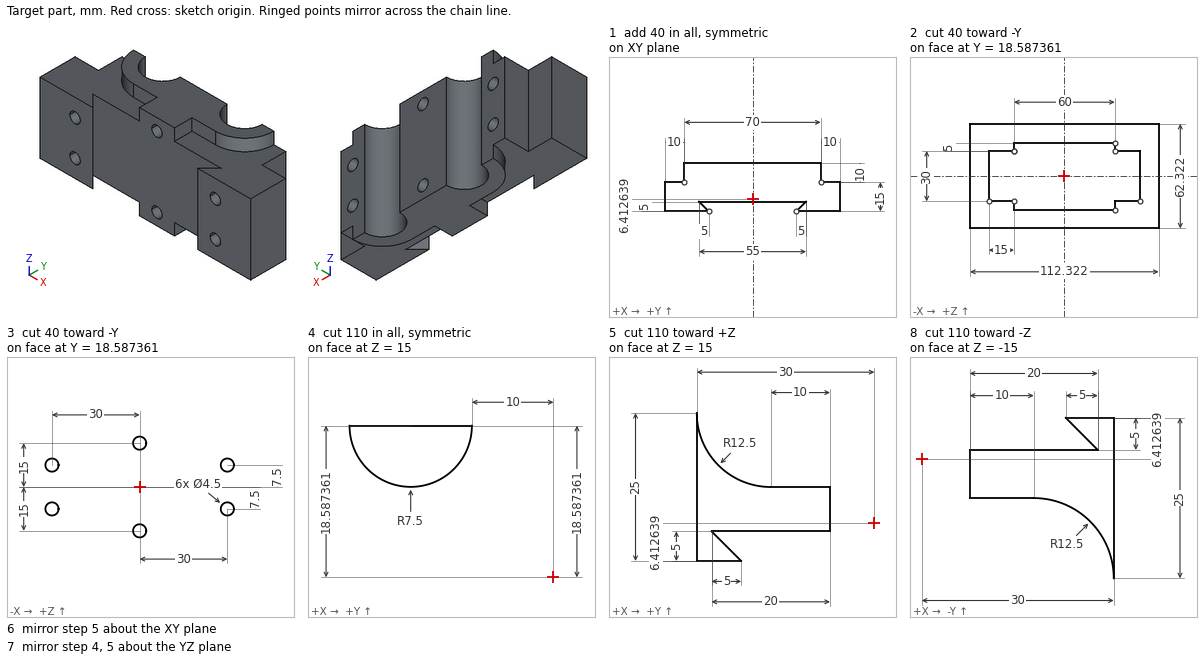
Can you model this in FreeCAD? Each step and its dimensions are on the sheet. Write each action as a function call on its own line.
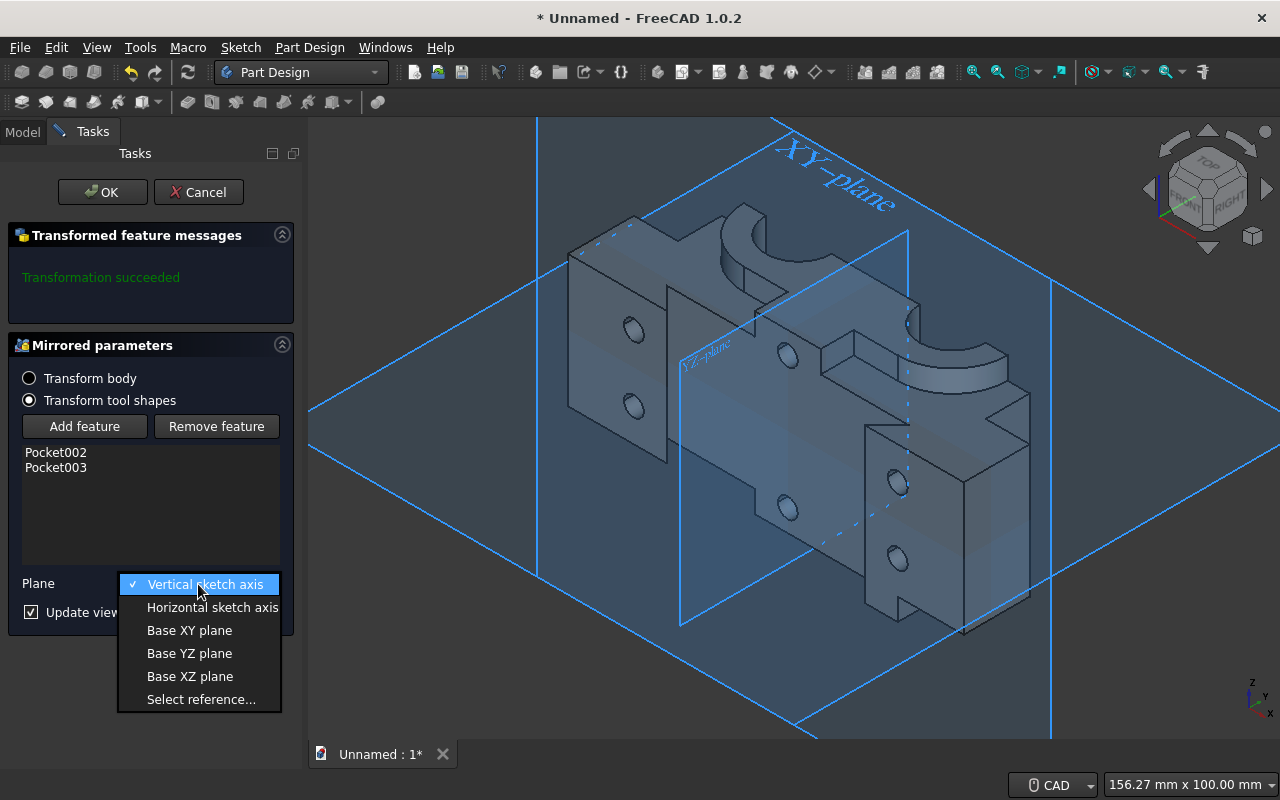
click(198, 654)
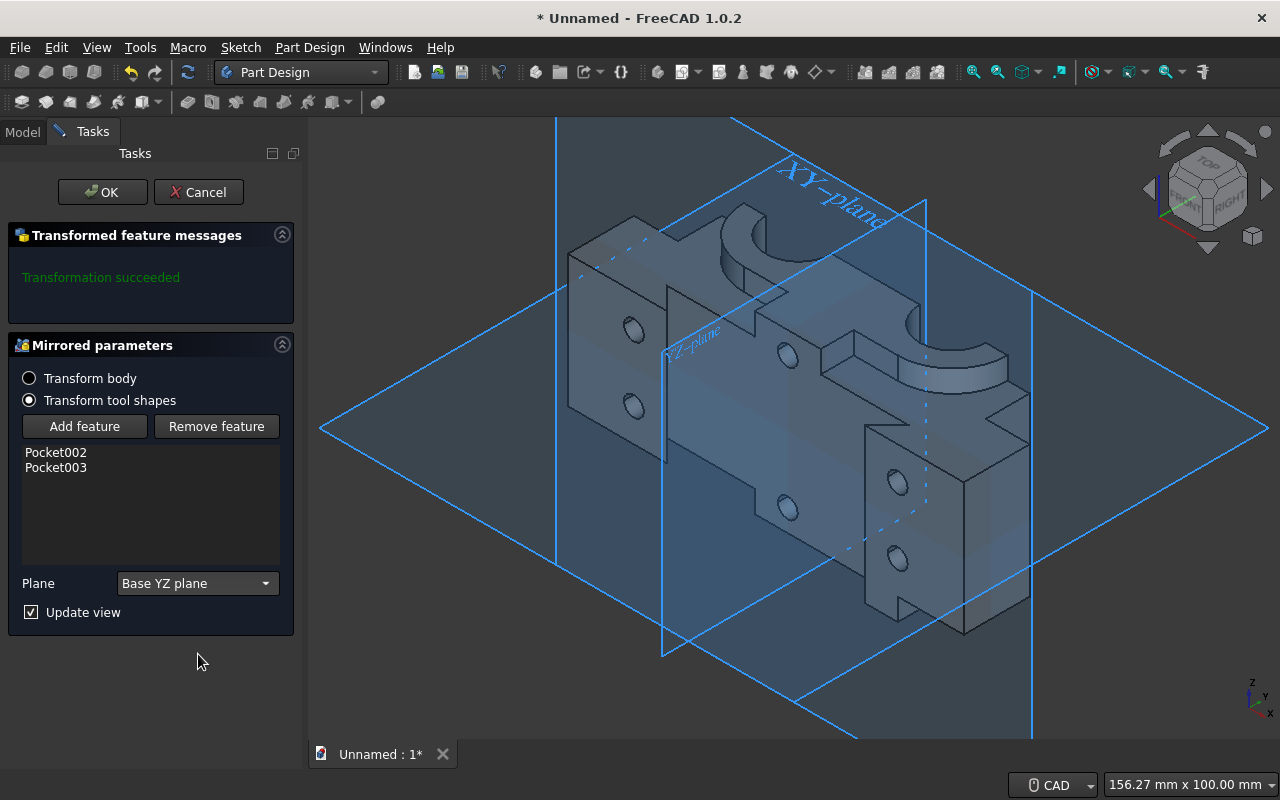
click(103, 192)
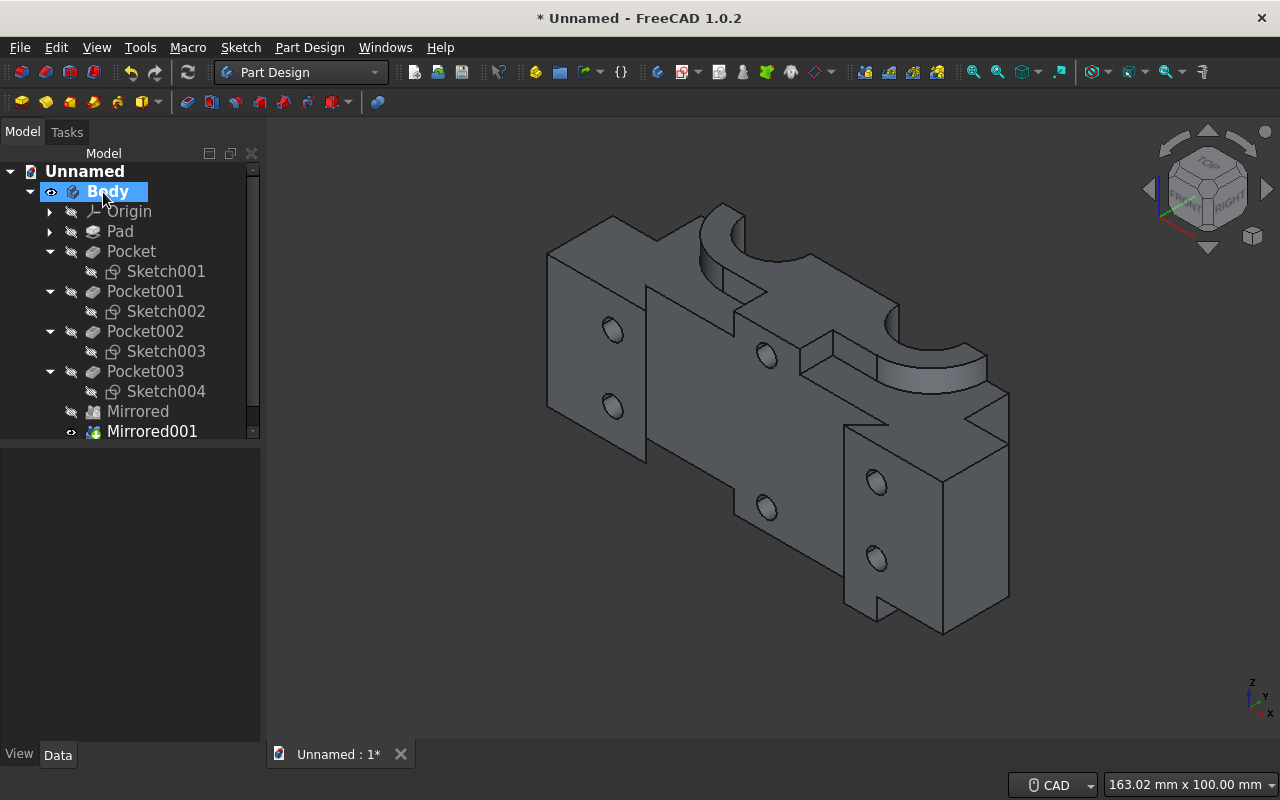
key(5)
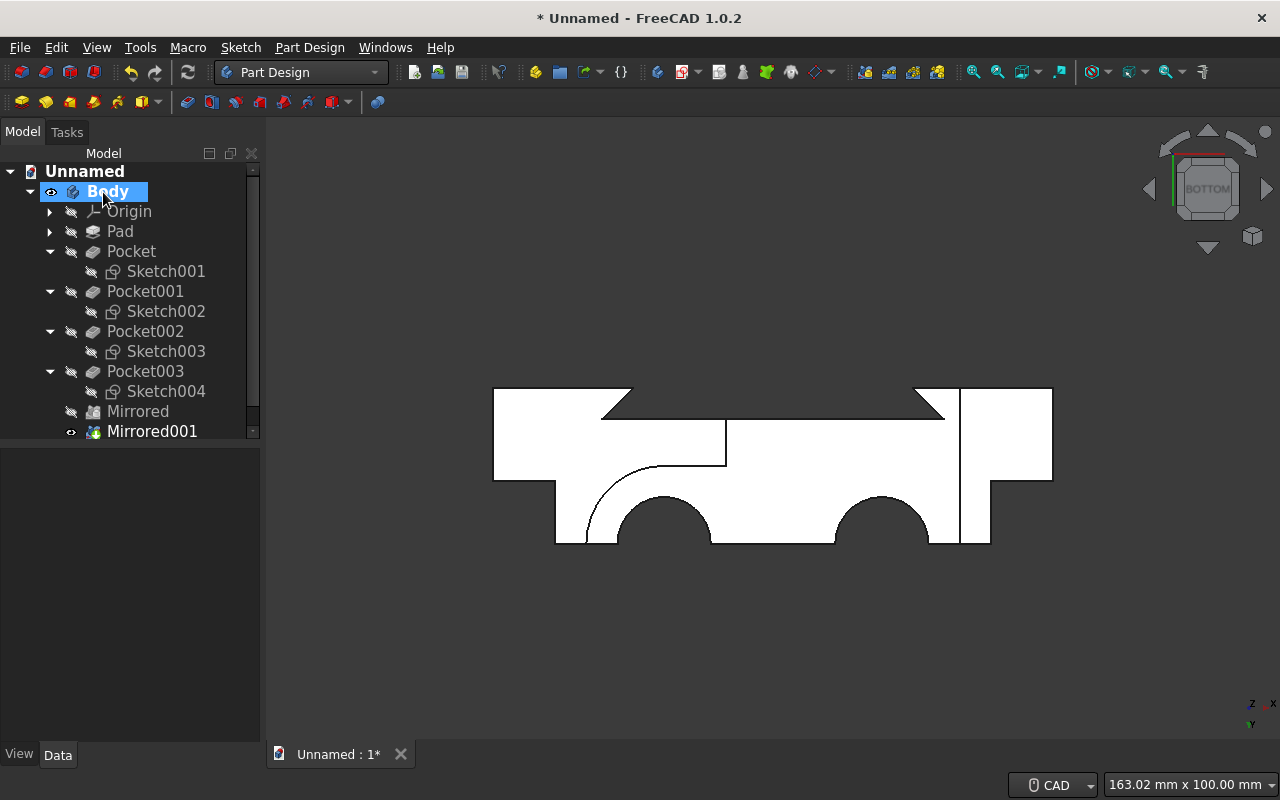
click(543, 443)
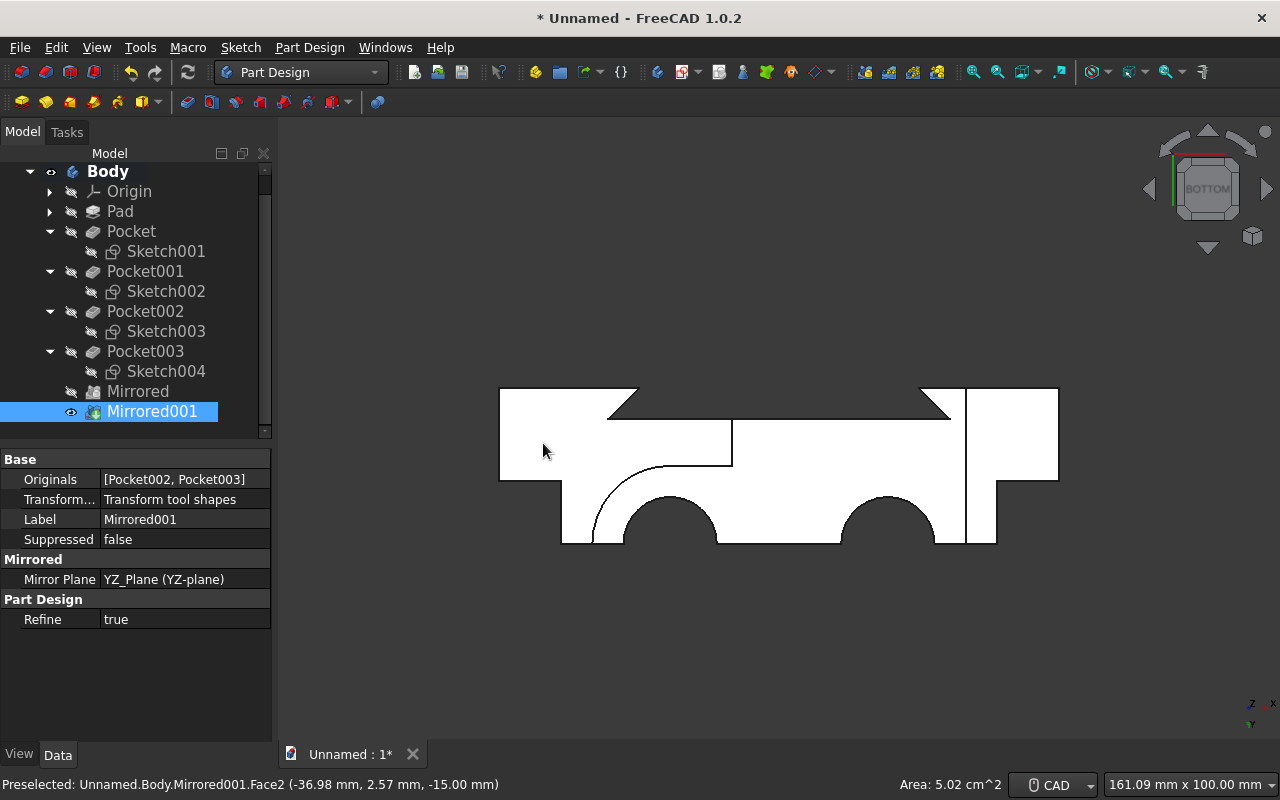
click(682, 72)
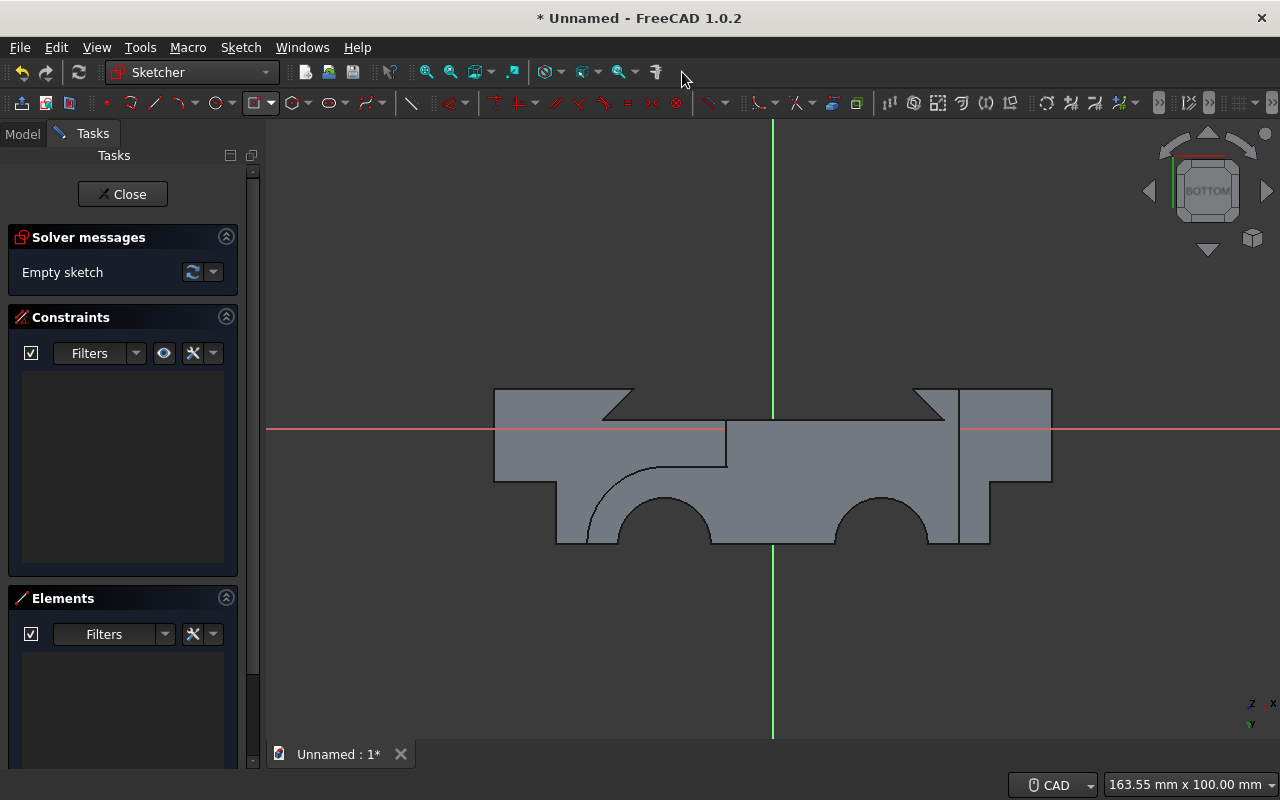
scroll(960, 489, up, 5)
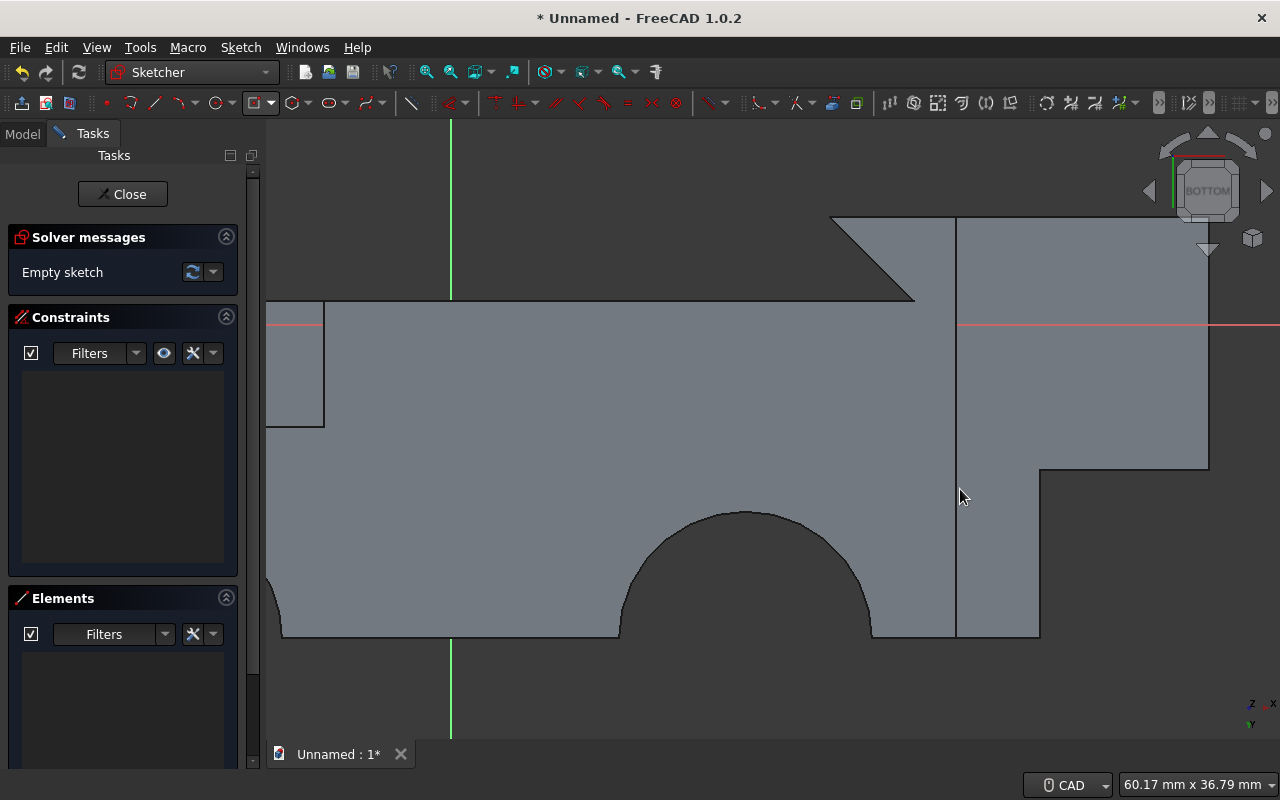
key(g)
key(m)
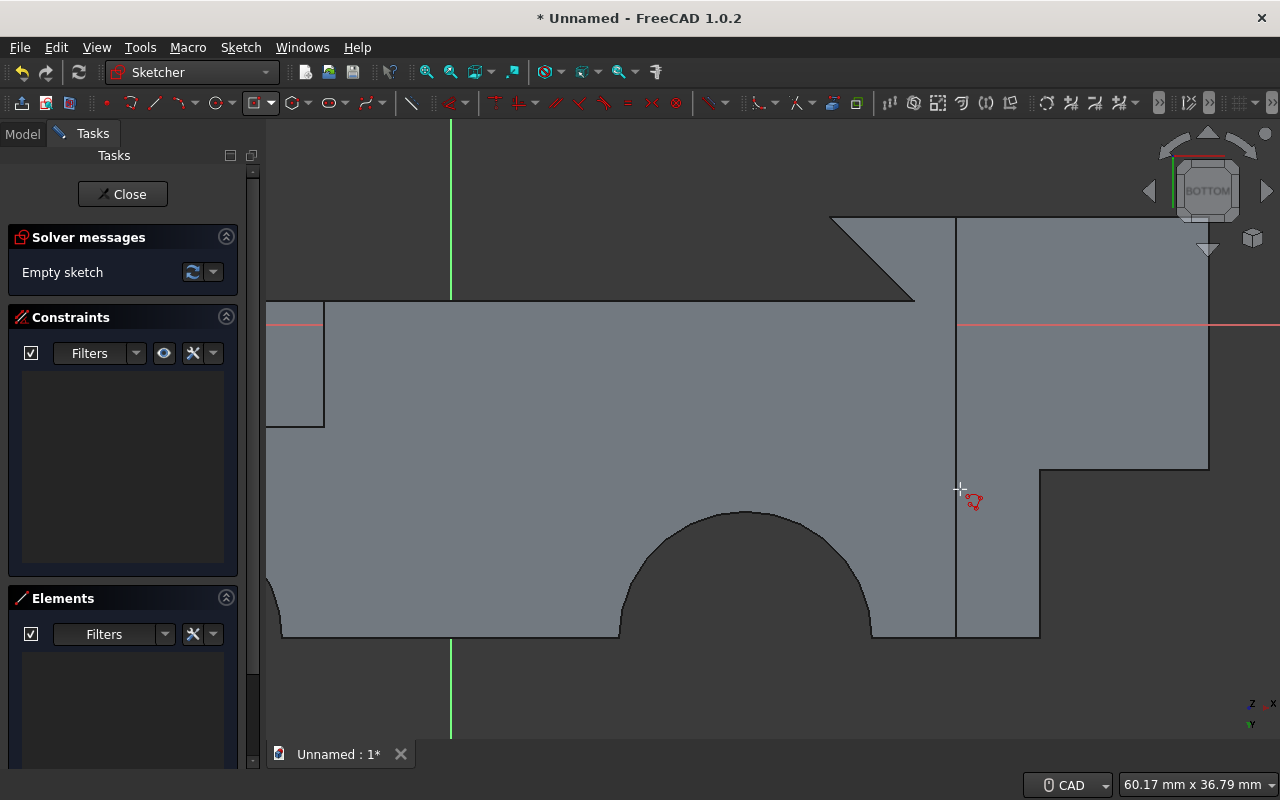
click(956, 638)
click(956, 217)
click(830, 217)
click(914, 301)
click(577, 301)
click(577, 427)
click(745, 427)
right_click(745, 427)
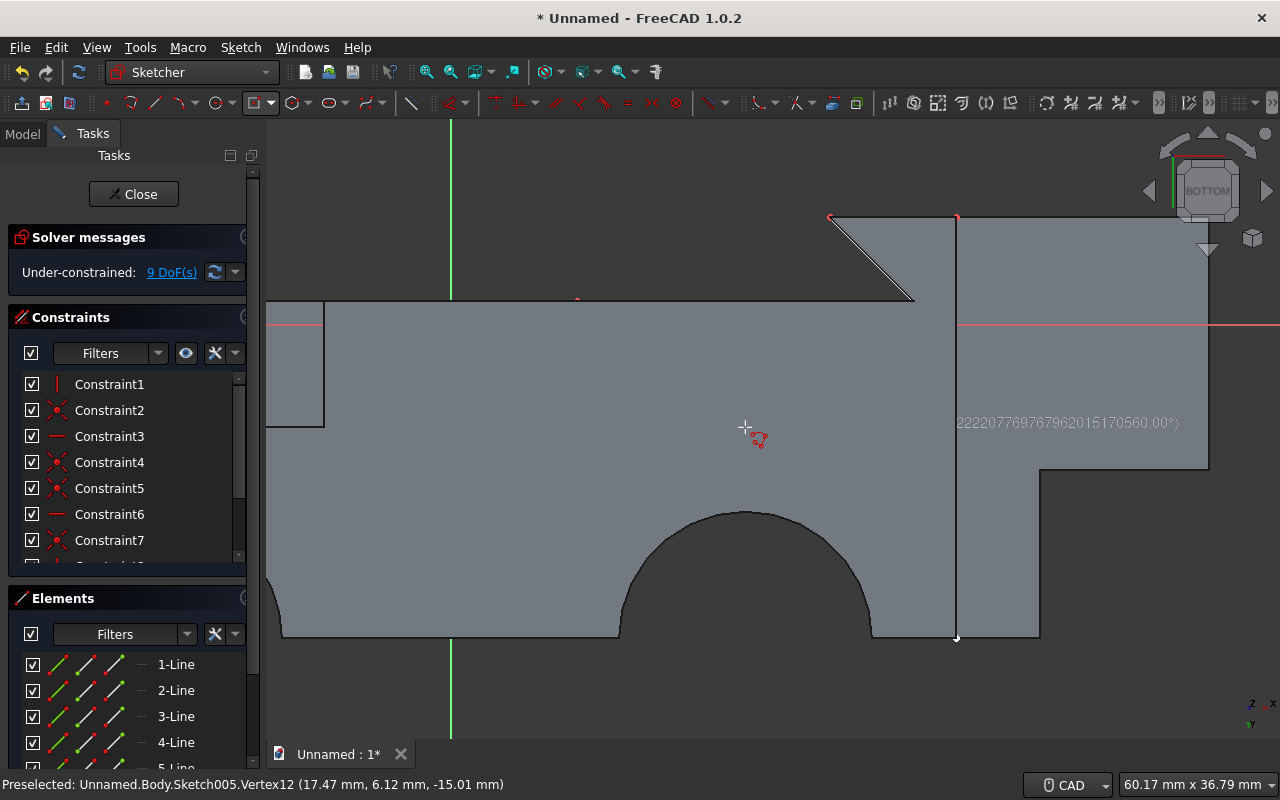
click(180, 104)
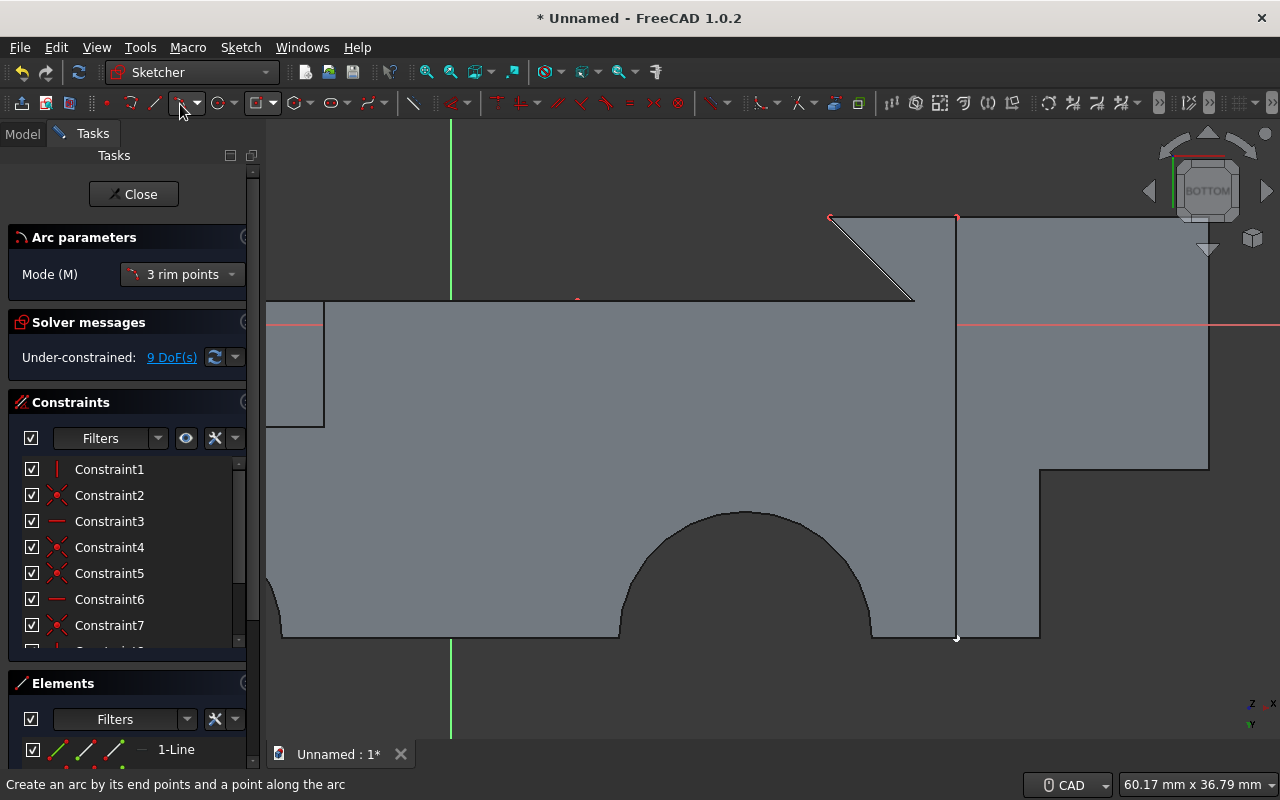
click(745, 428)
click(956, 639)
click(894, 489)
key(Escape)